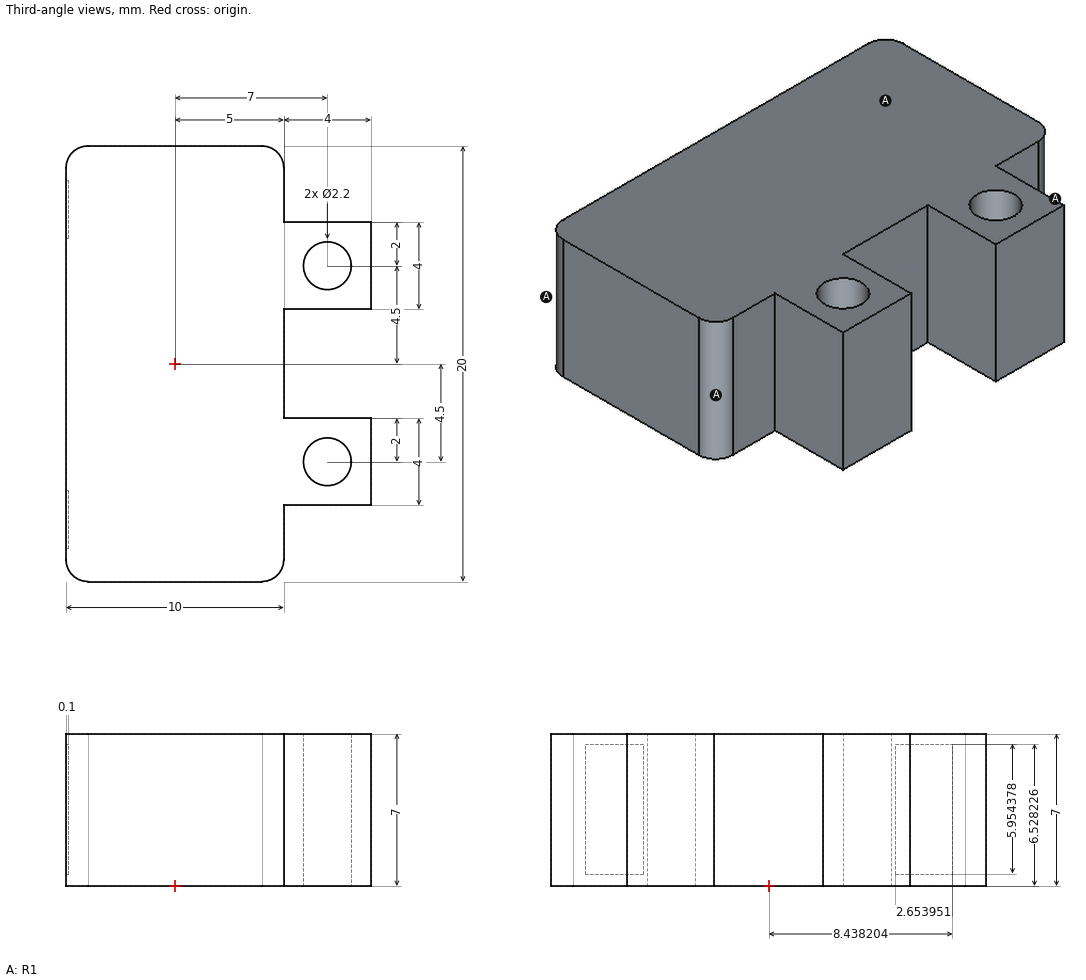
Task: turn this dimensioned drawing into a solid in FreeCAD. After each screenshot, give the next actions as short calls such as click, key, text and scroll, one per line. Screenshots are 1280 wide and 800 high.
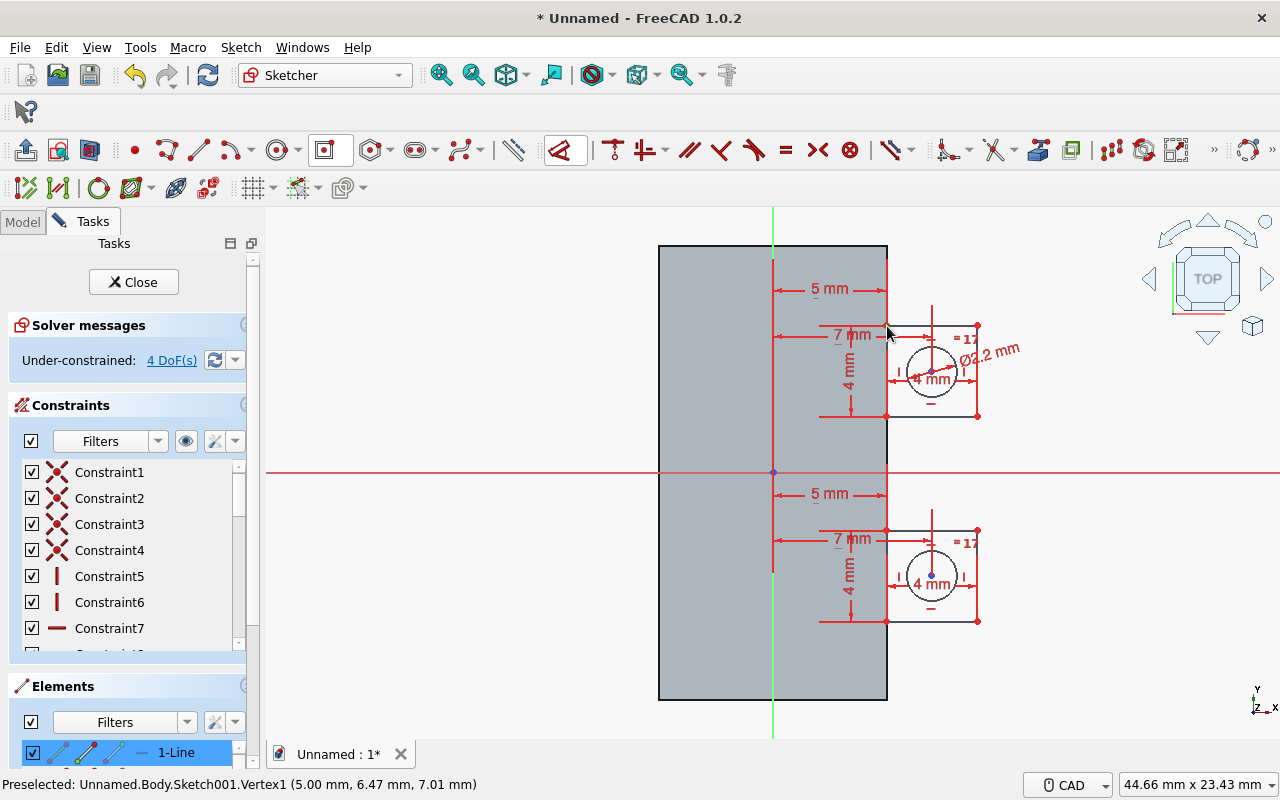
click(932, 372)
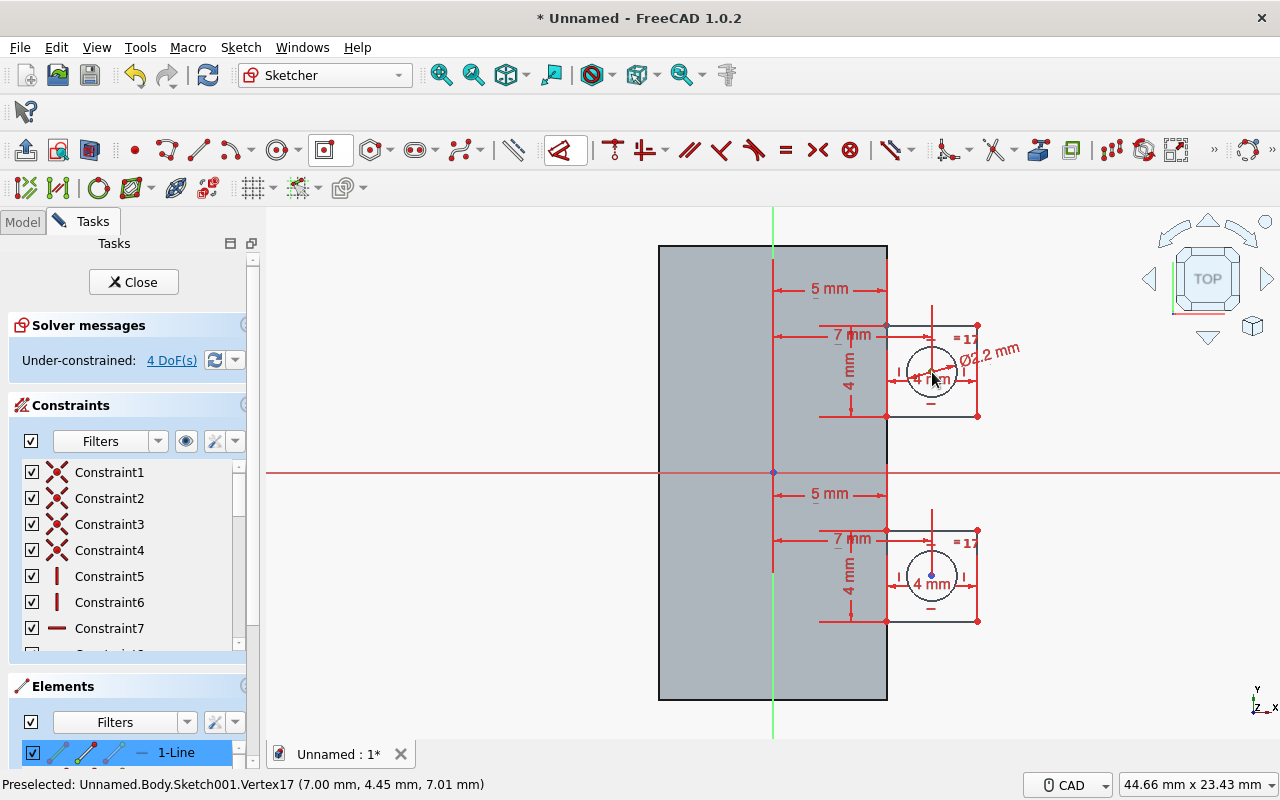
key(i)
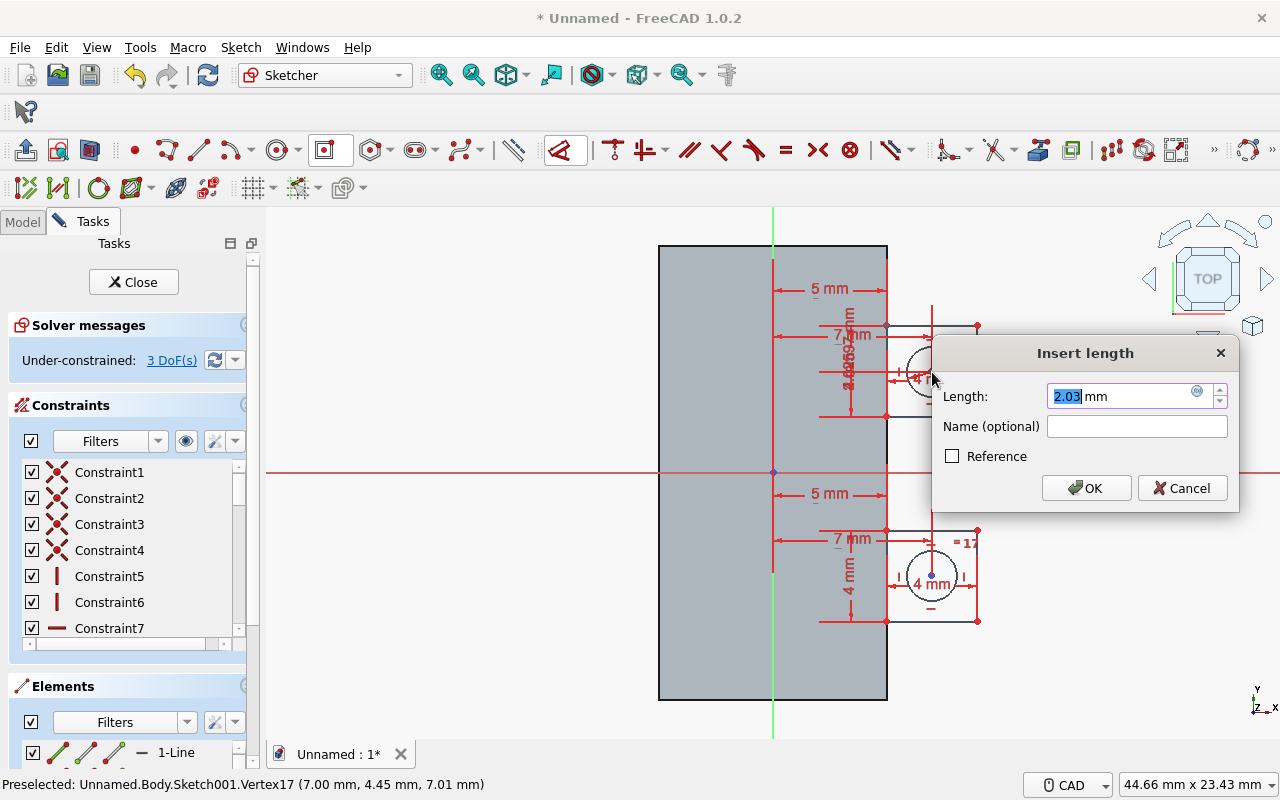
text(2)
key(Return)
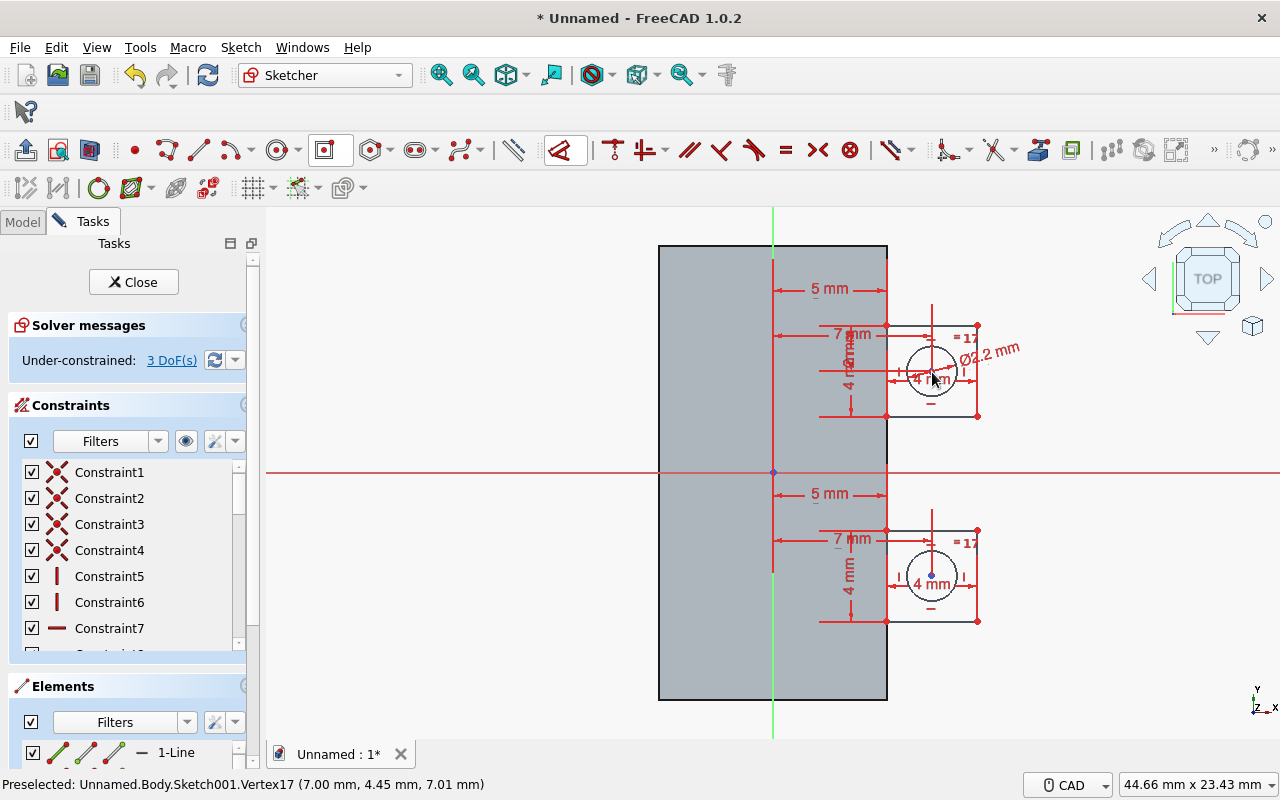
click(887, 531)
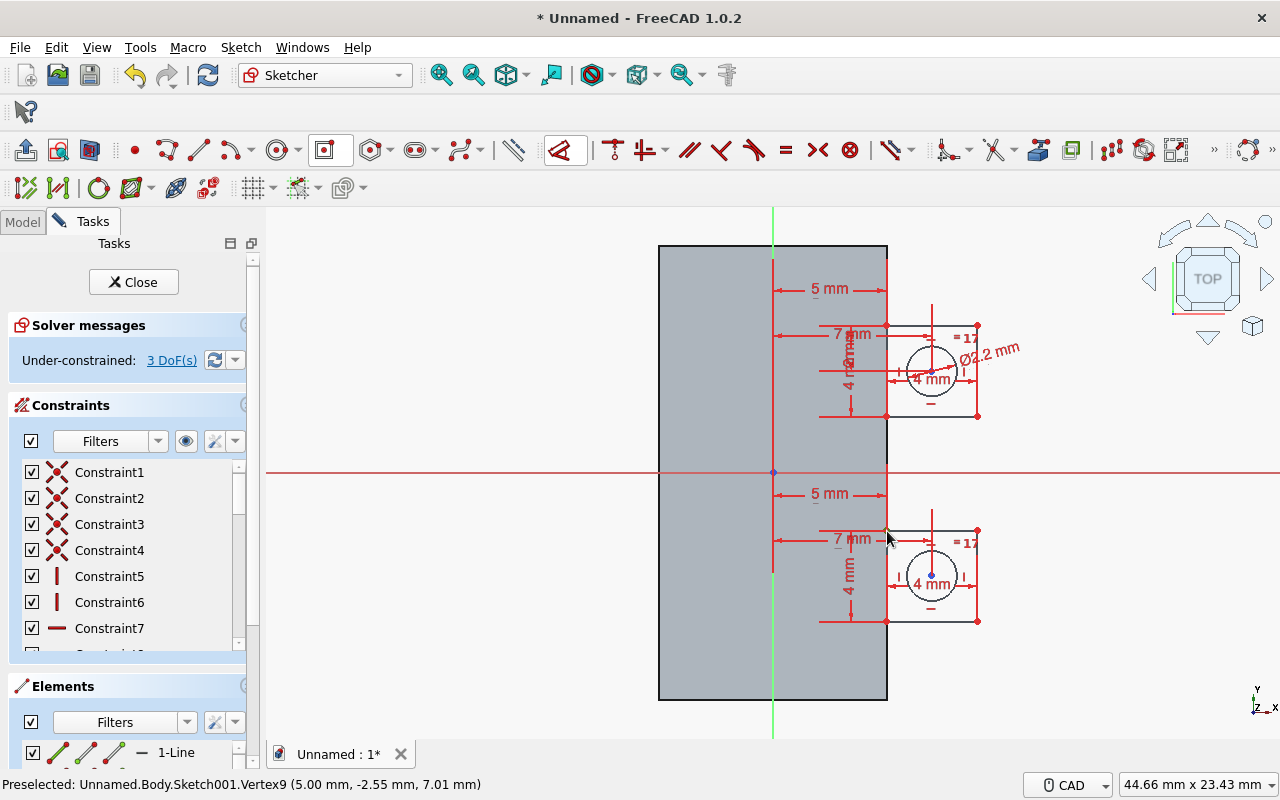
click(932, 576)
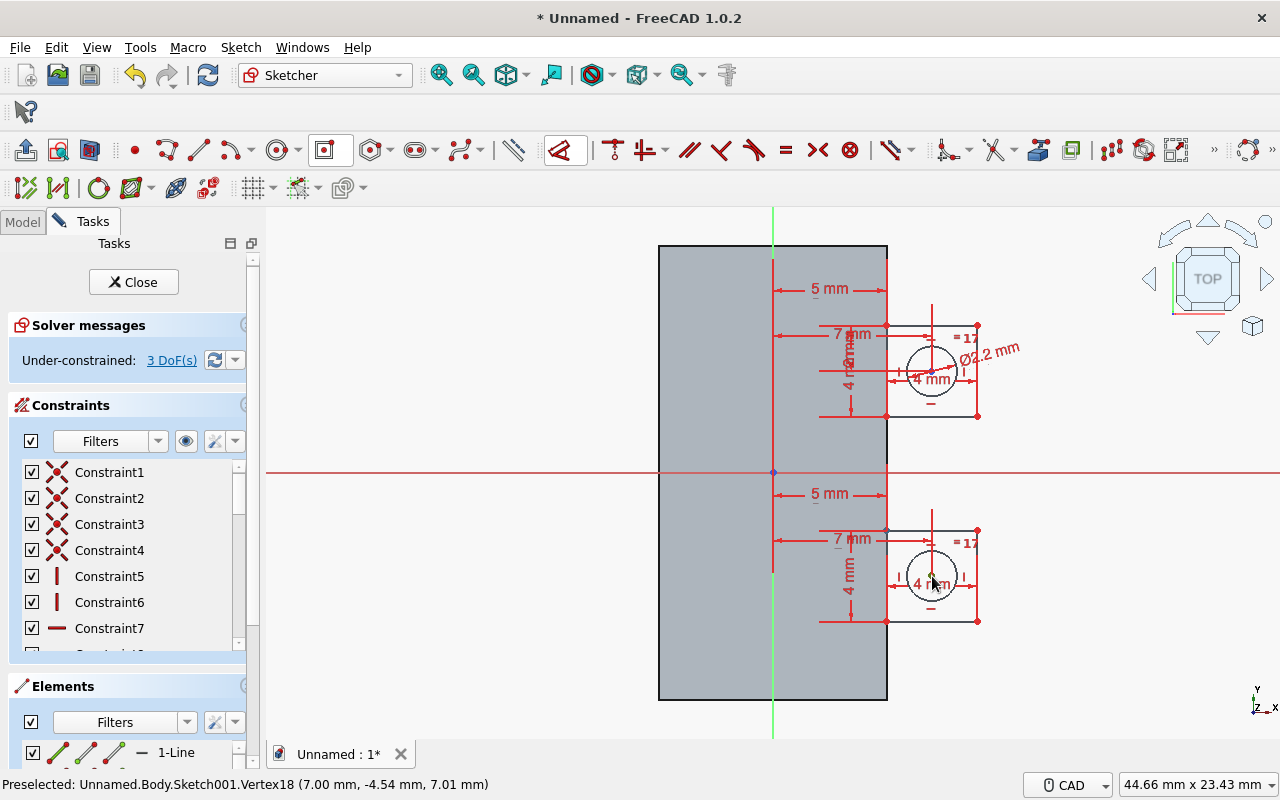
key(i)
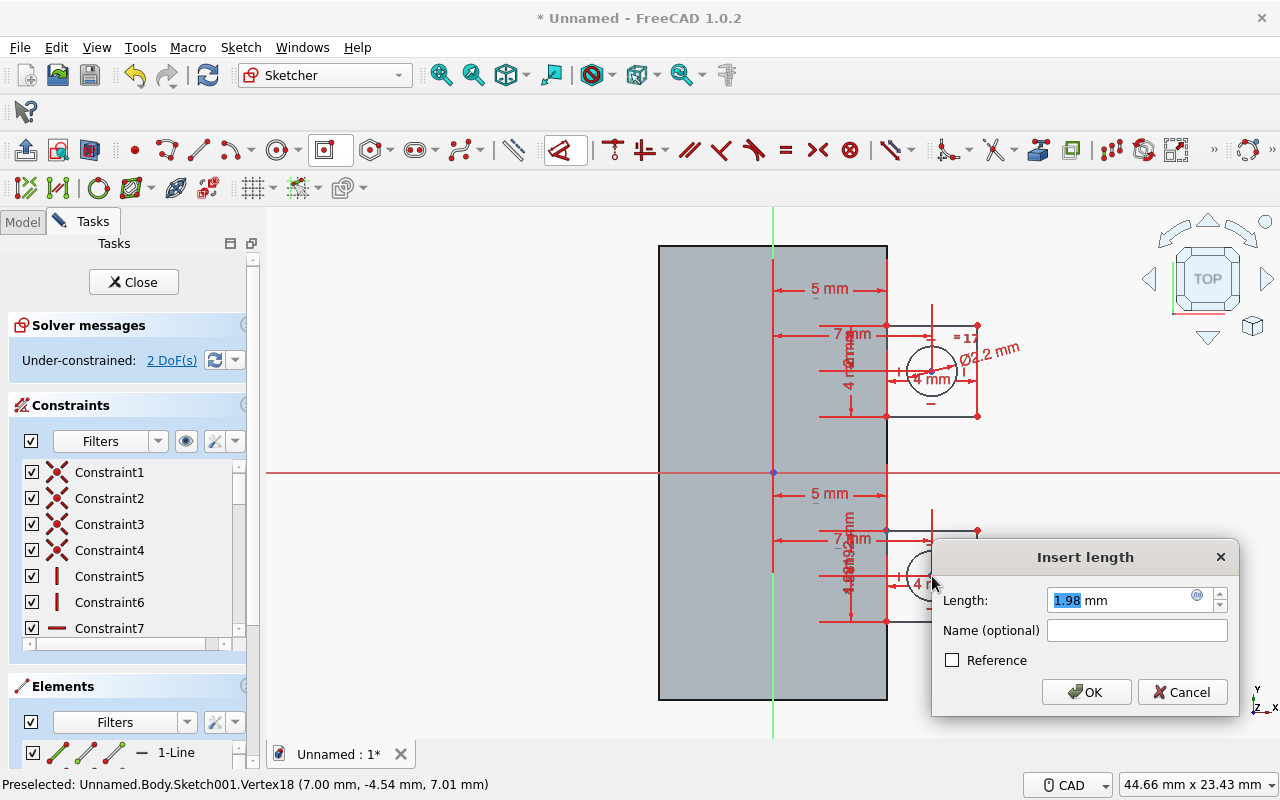
text(2)
key(Return)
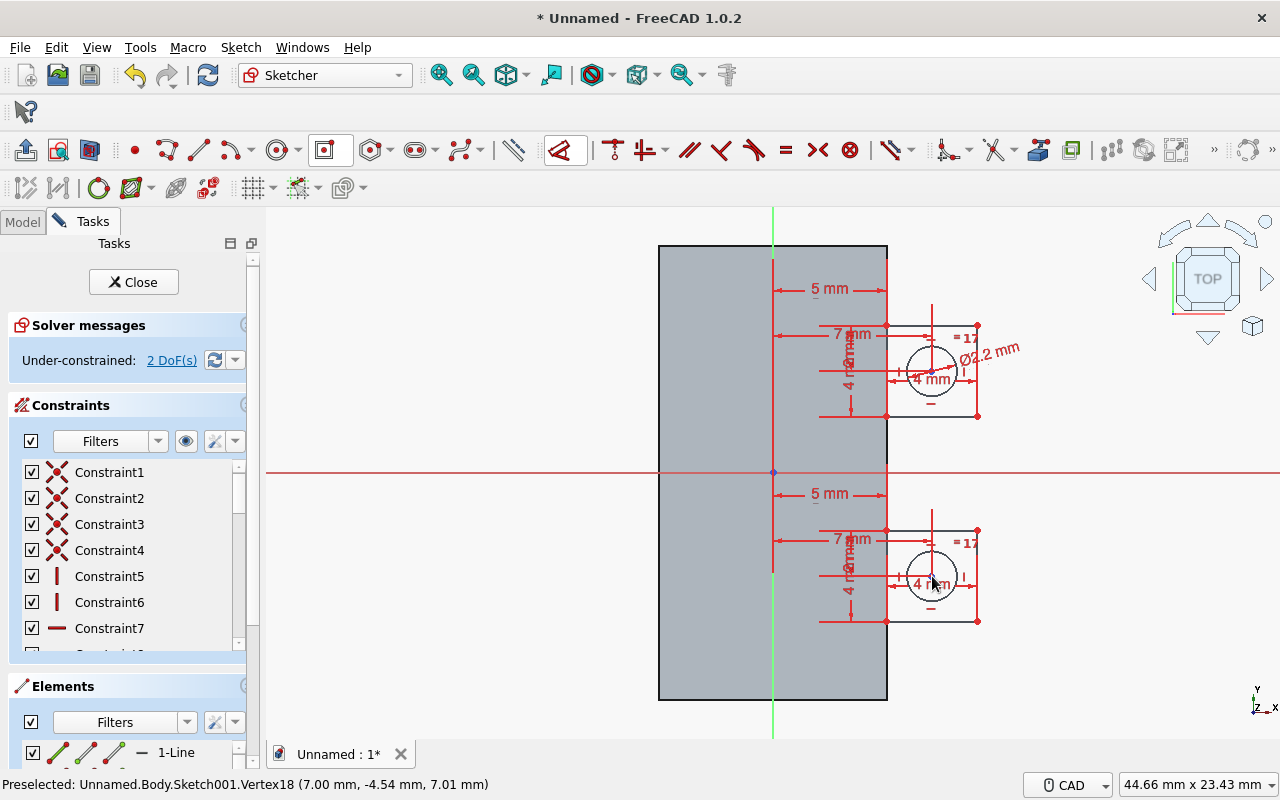
click(932, 371)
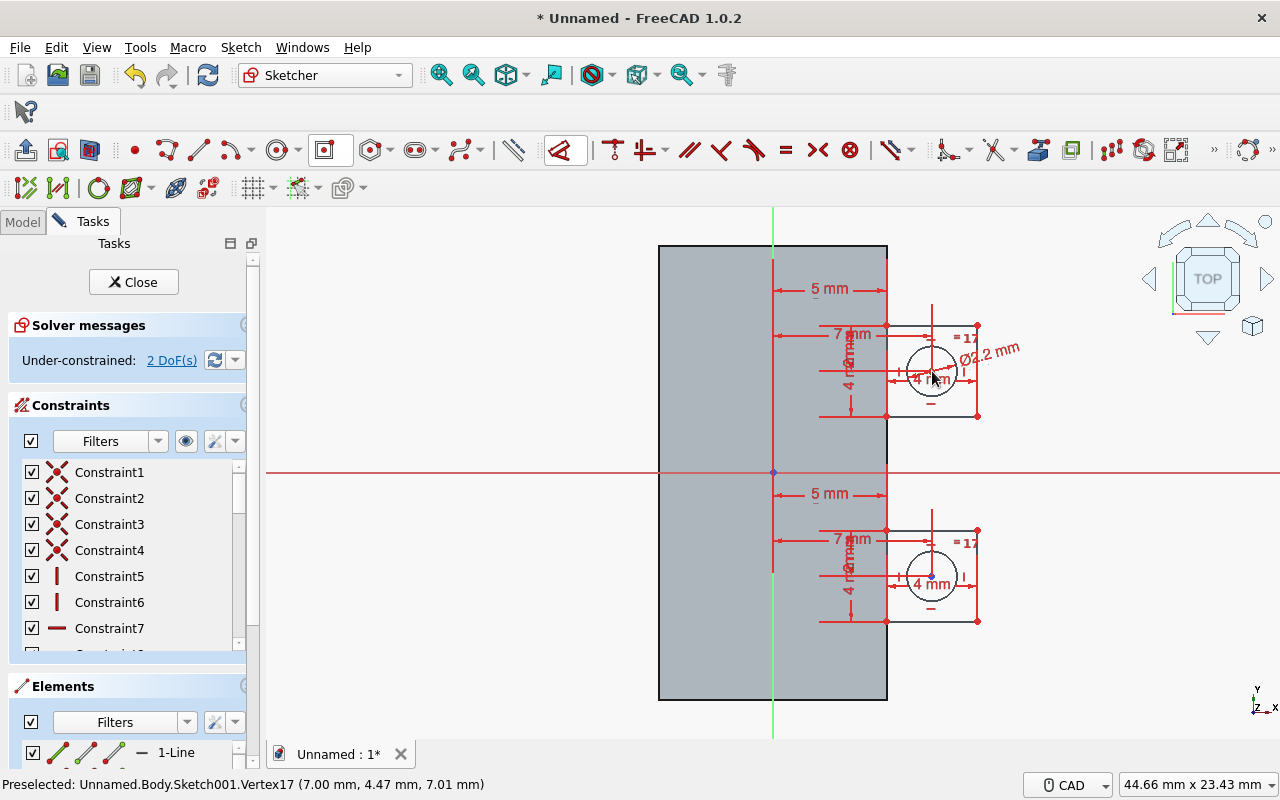
key(i)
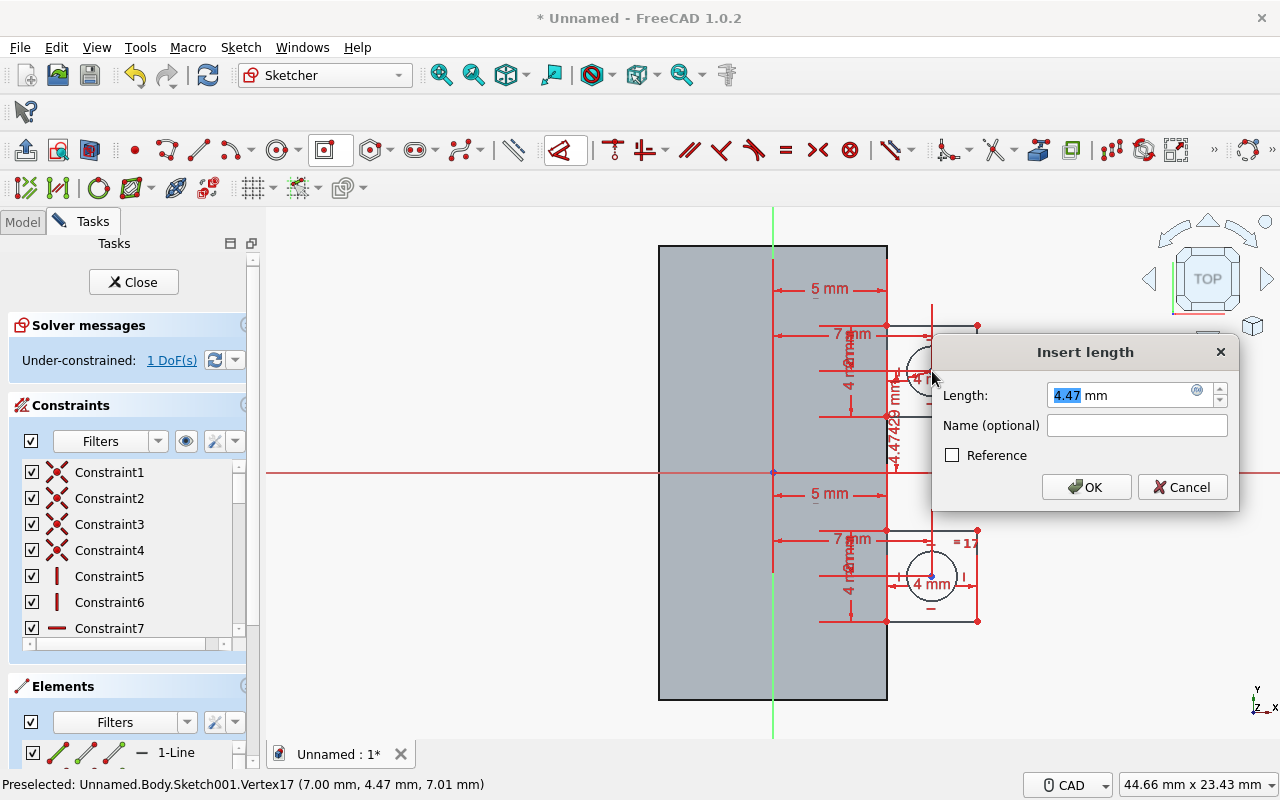
text(4.5)
key(Return)